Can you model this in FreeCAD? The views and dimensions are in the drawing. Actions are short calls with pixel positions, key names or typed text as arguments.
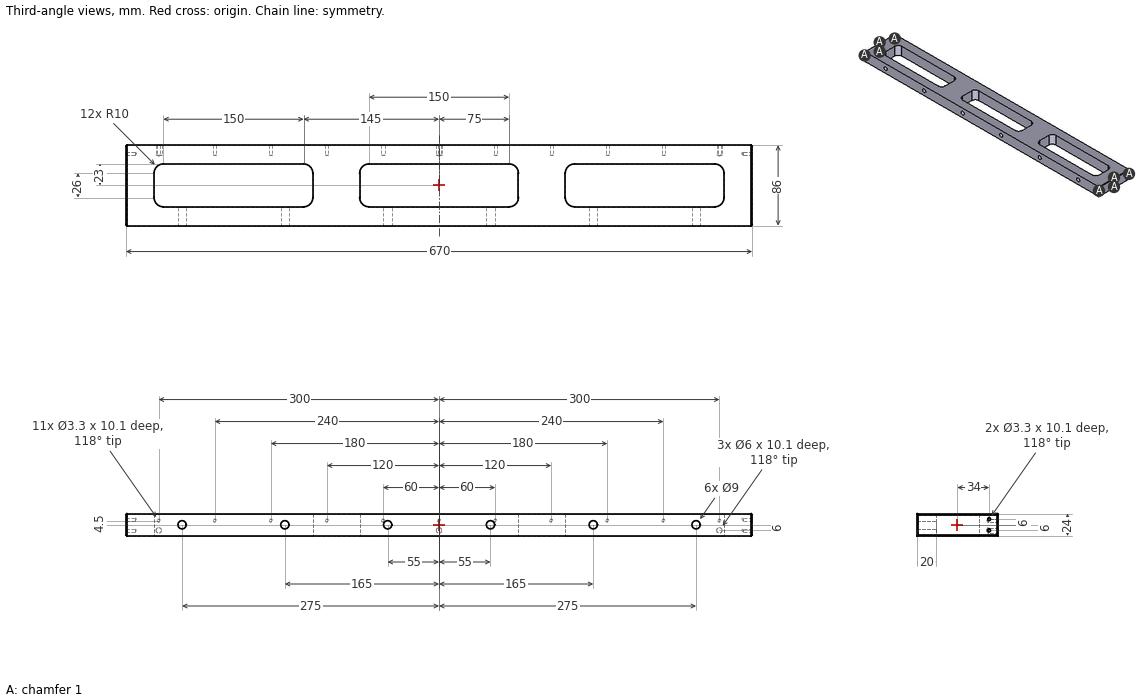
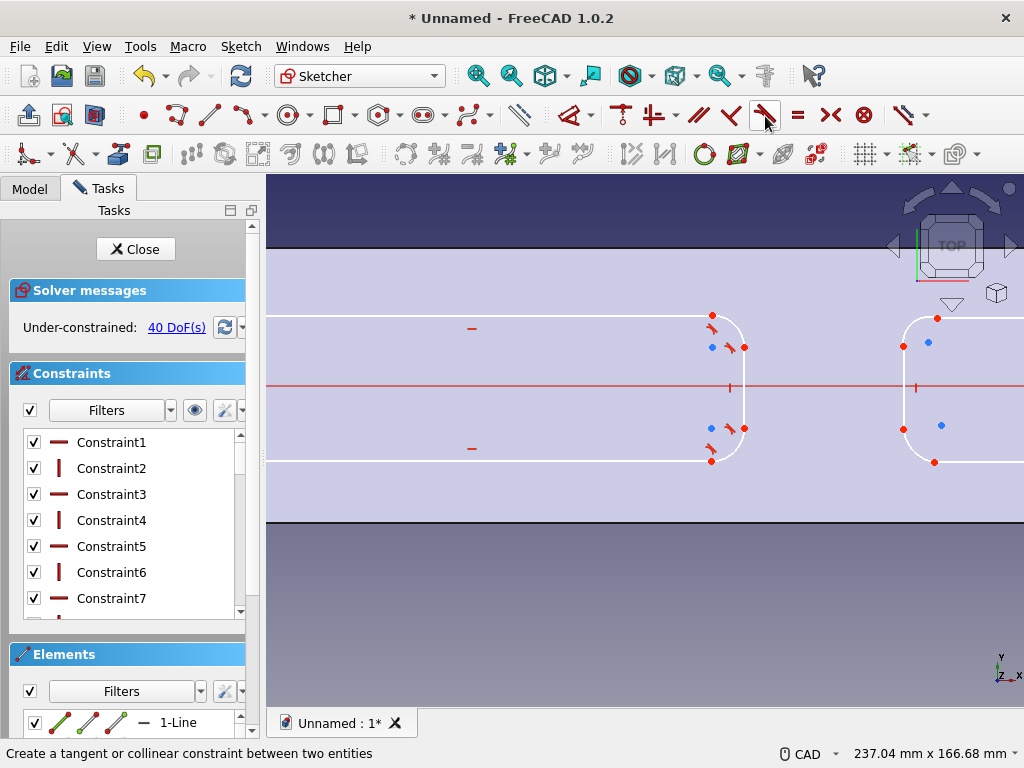
scroll(425, 454, down, 8)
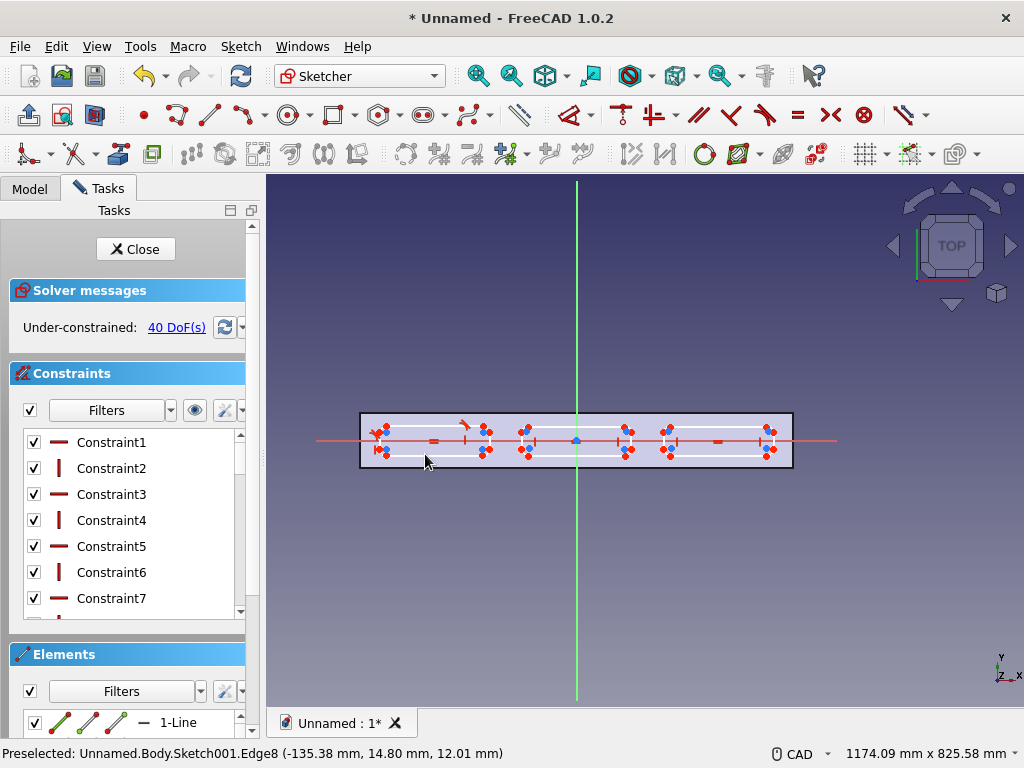
click(596, 427)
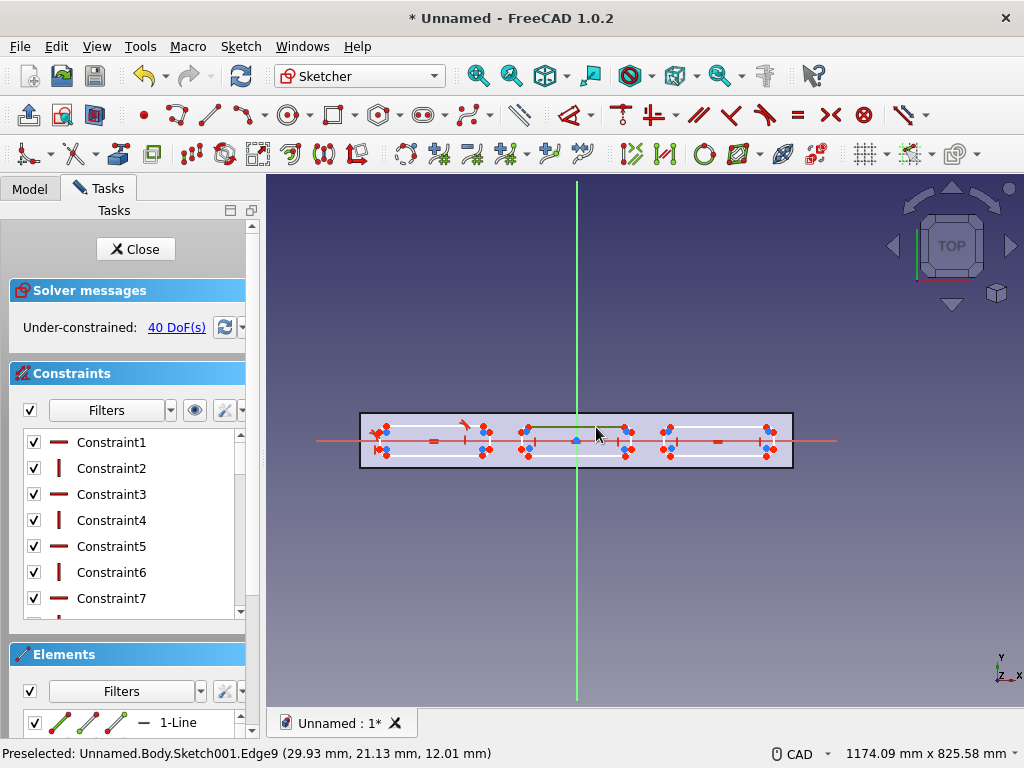
scroll(524, 428, up, 5)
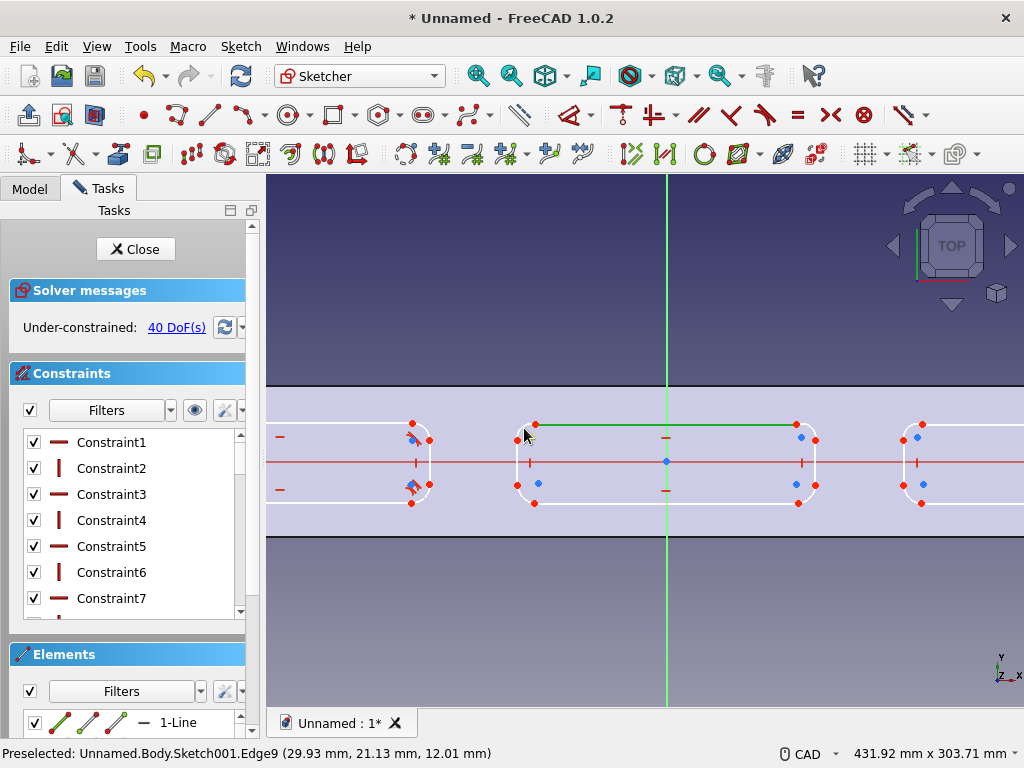
click(522, 427)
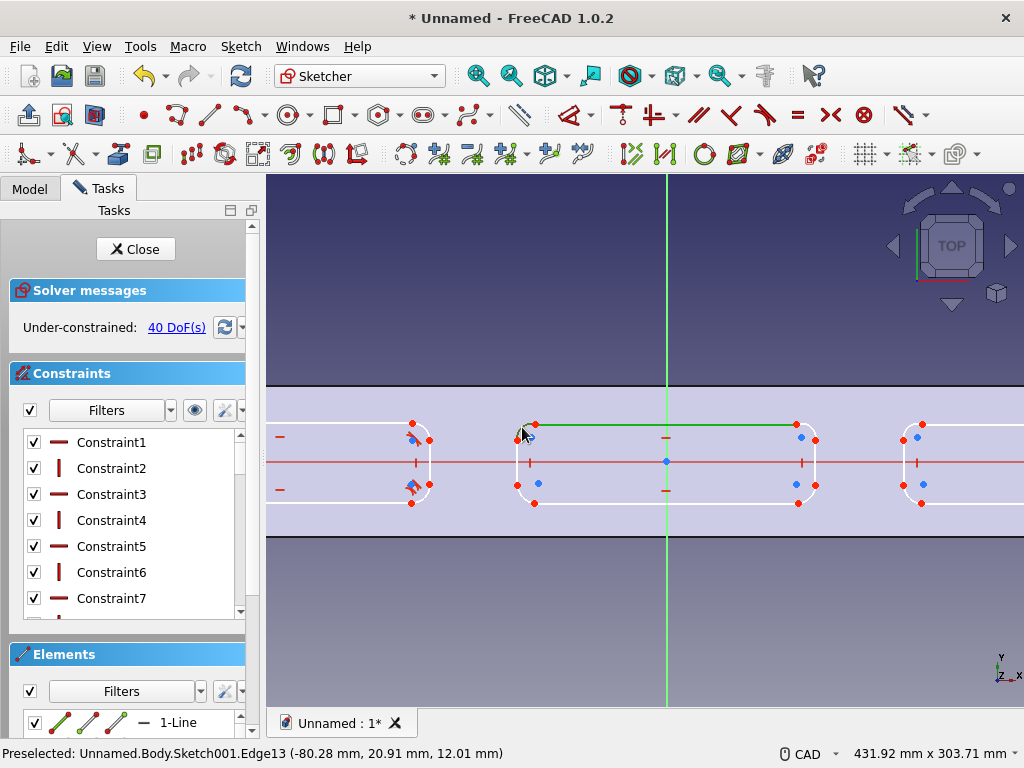
click(765, 116)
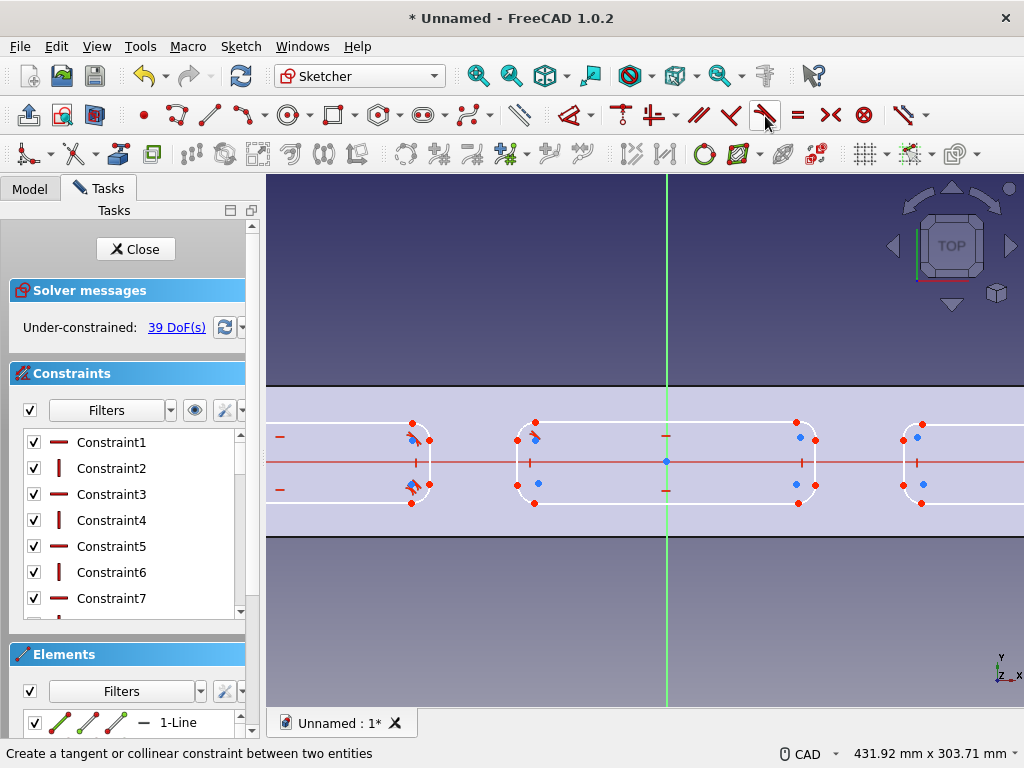
click(719, 422)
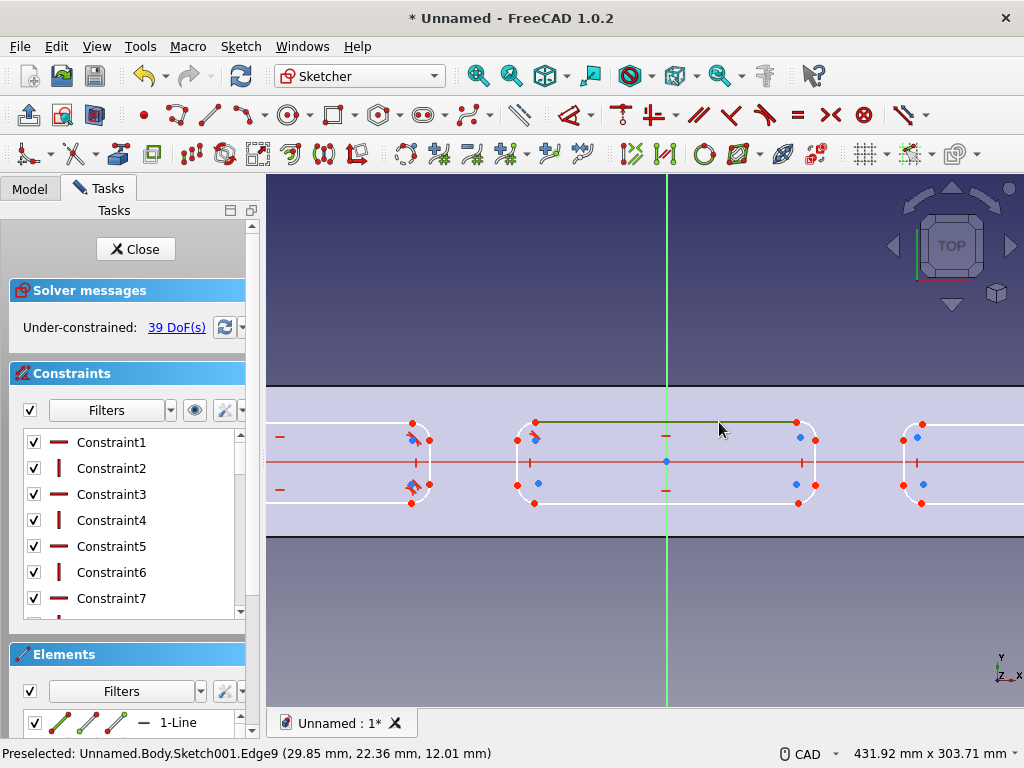
click(811, 426)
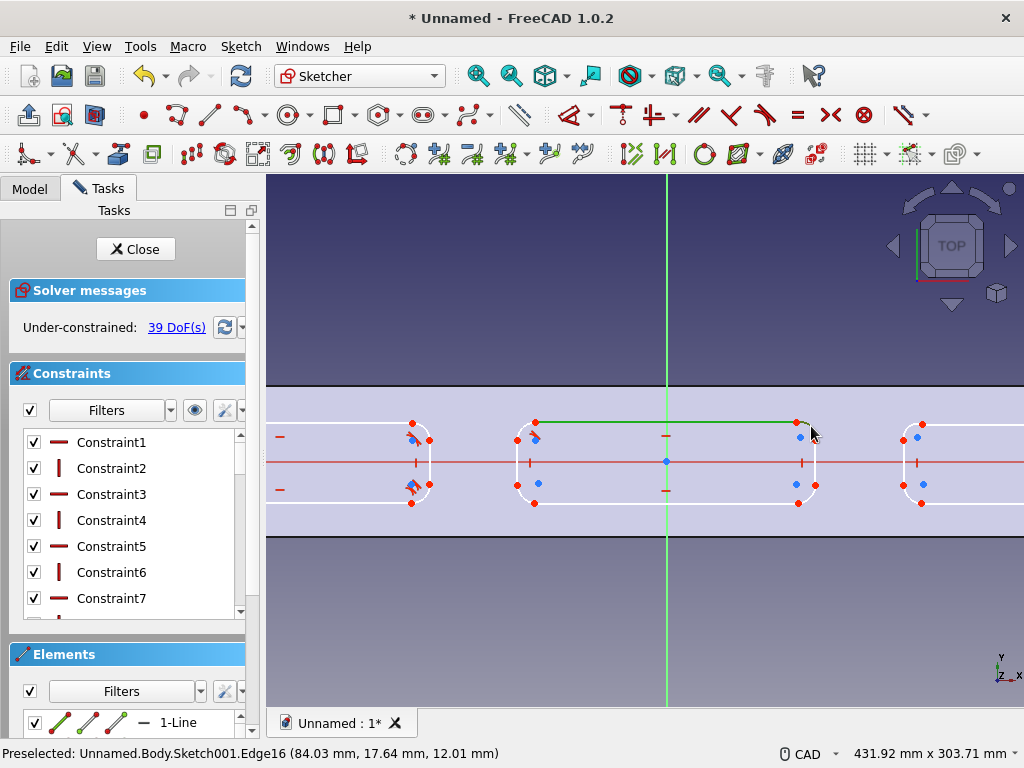
key(t)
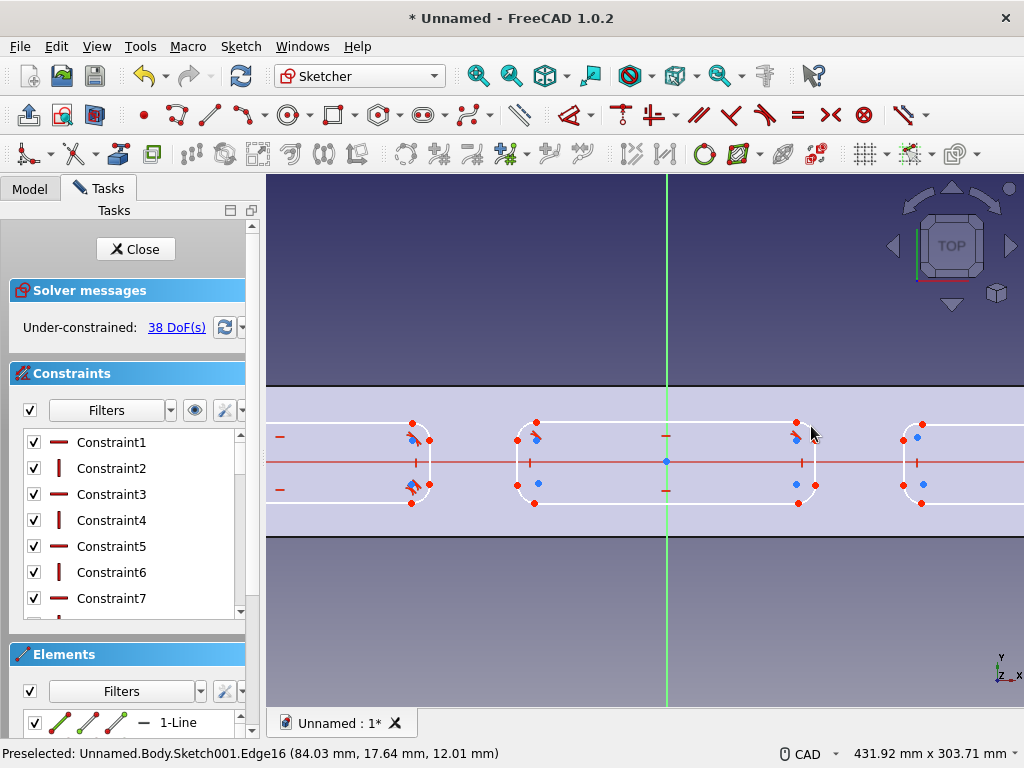
scroll(517, 472, up, 2)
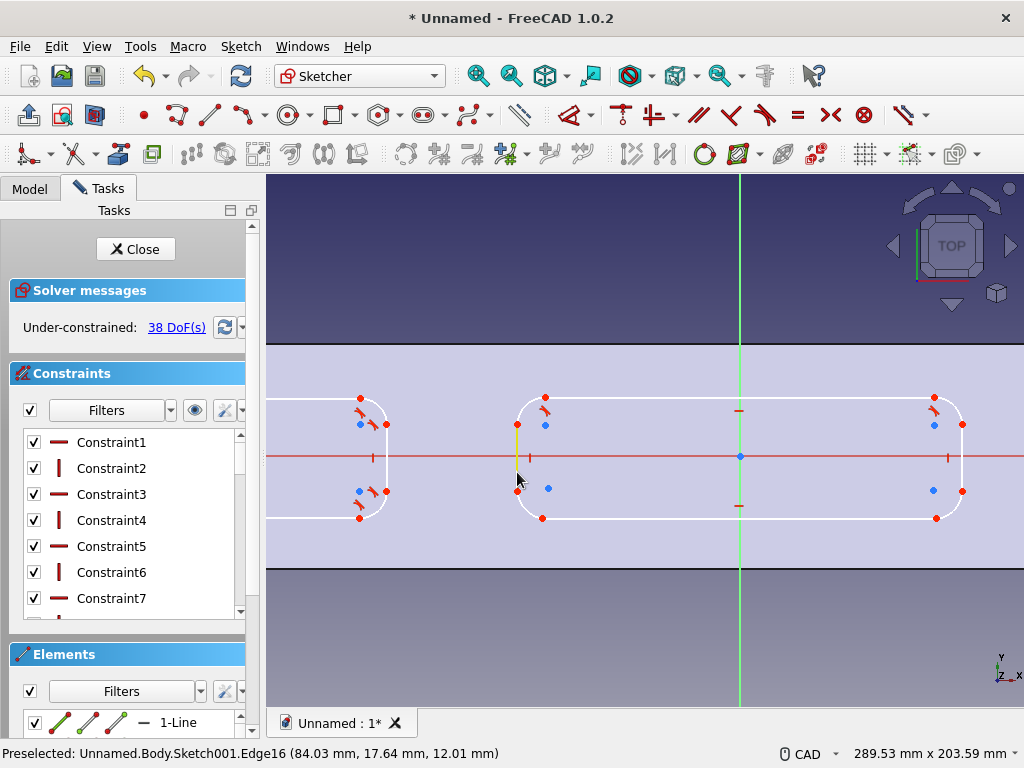
click(517, 471)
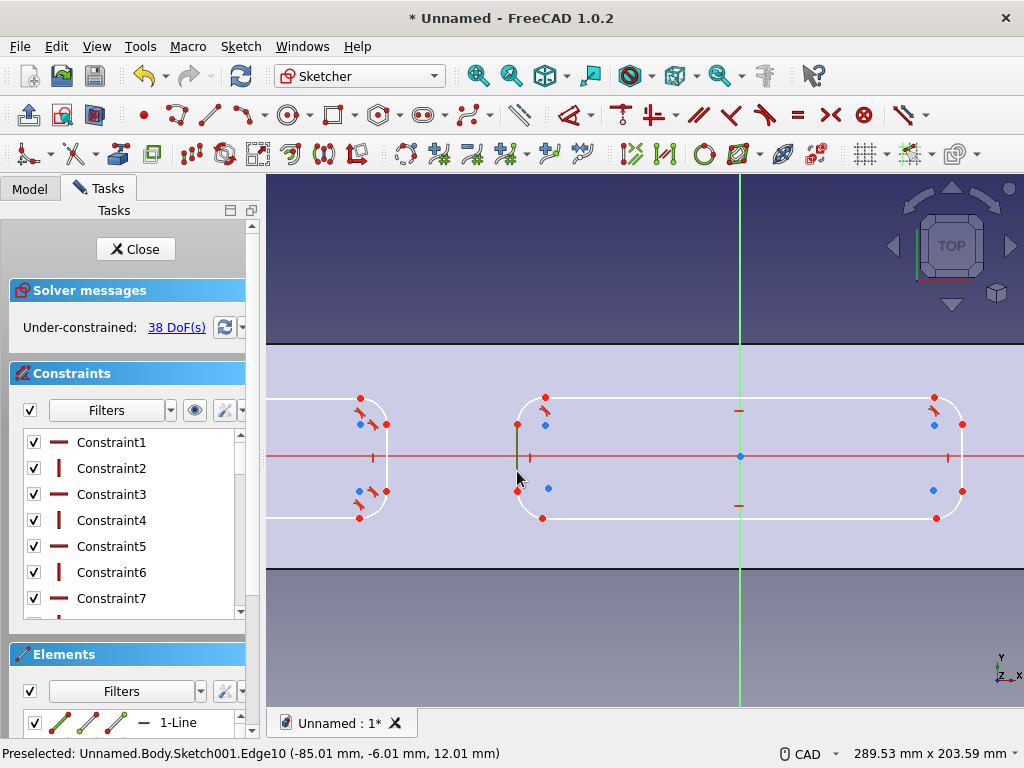
click(533, 400)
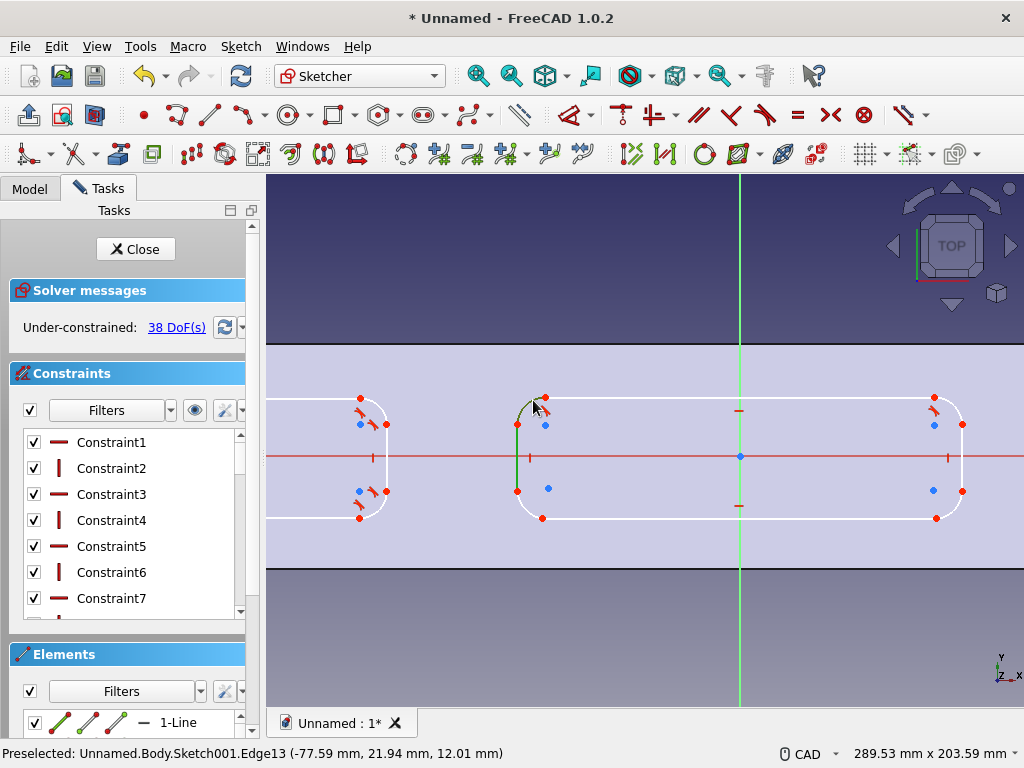
key(t)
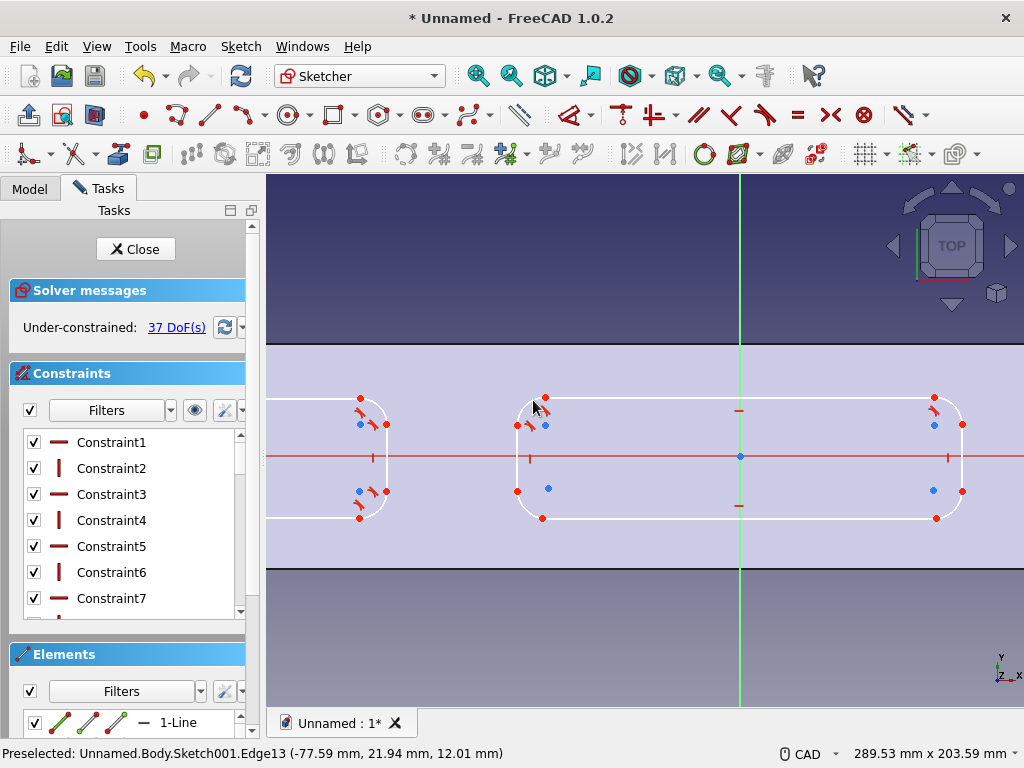
scroll(517, 445, up, 2)